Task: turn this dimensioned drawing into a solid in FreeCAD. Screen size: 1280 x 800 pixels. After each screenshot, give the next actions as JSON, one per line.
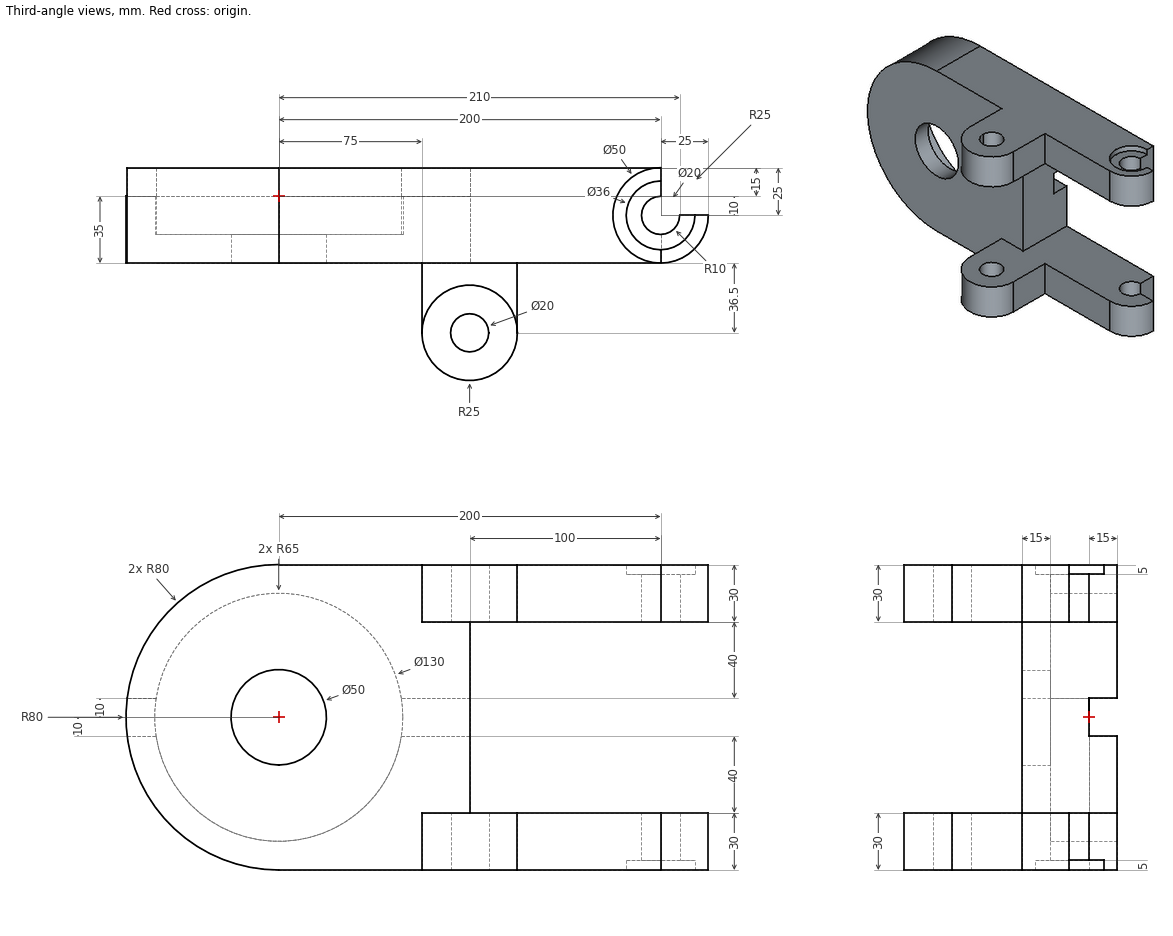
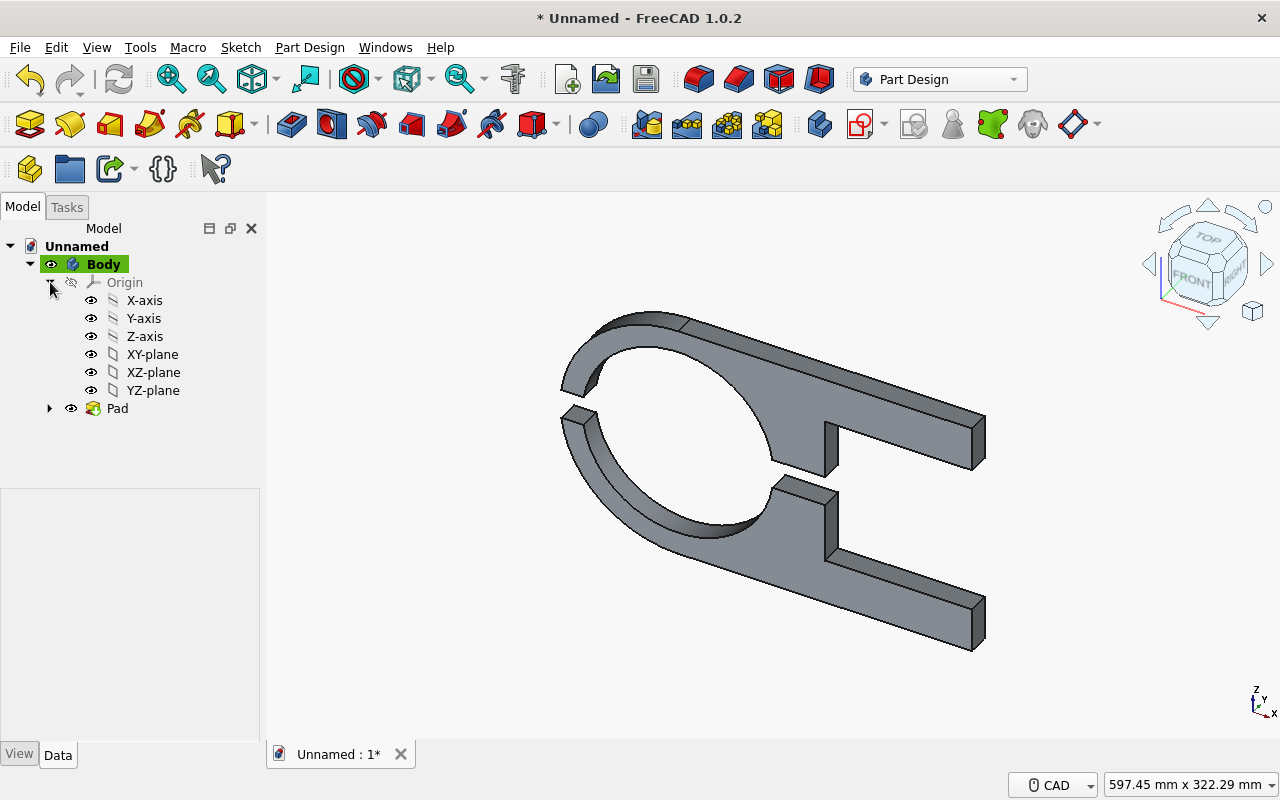
{"action": "left_click", "coordinate": [136, 372]}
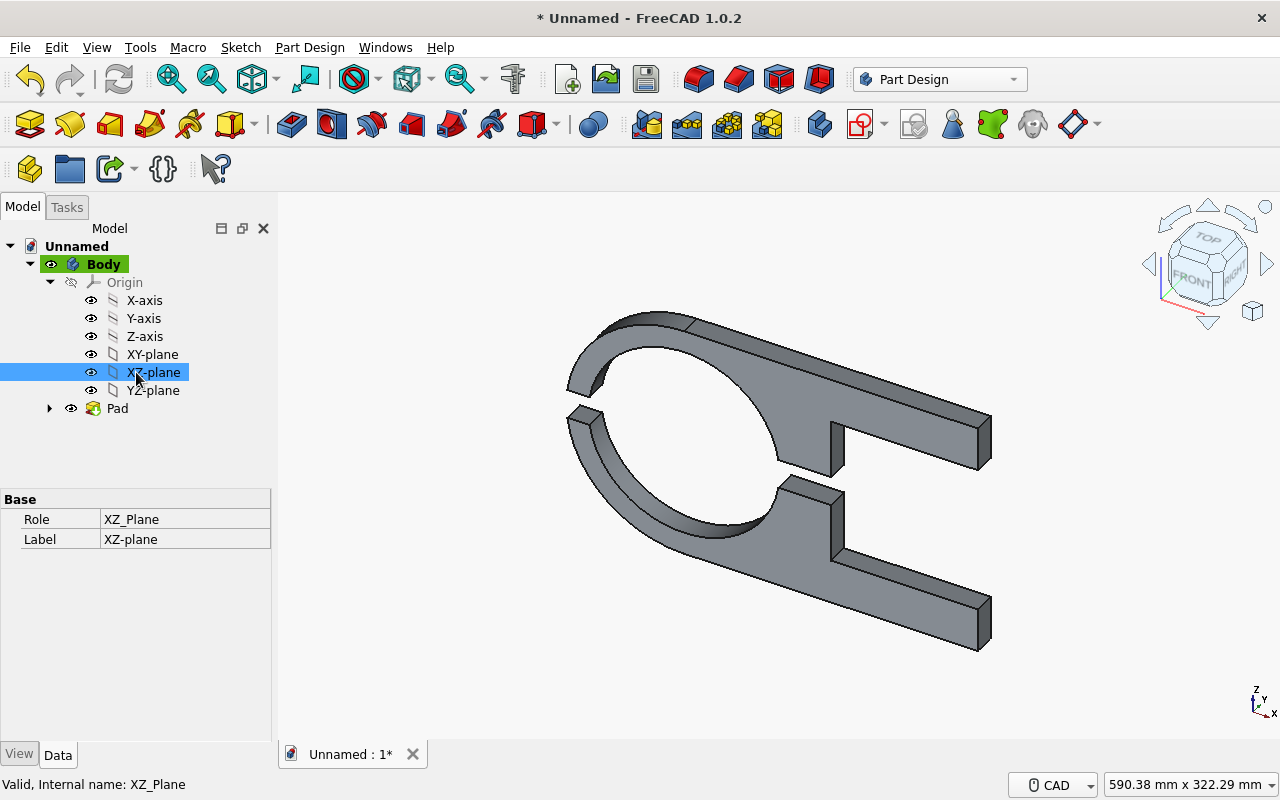
{"action": "left_click", "coordinate": [1074, 124]}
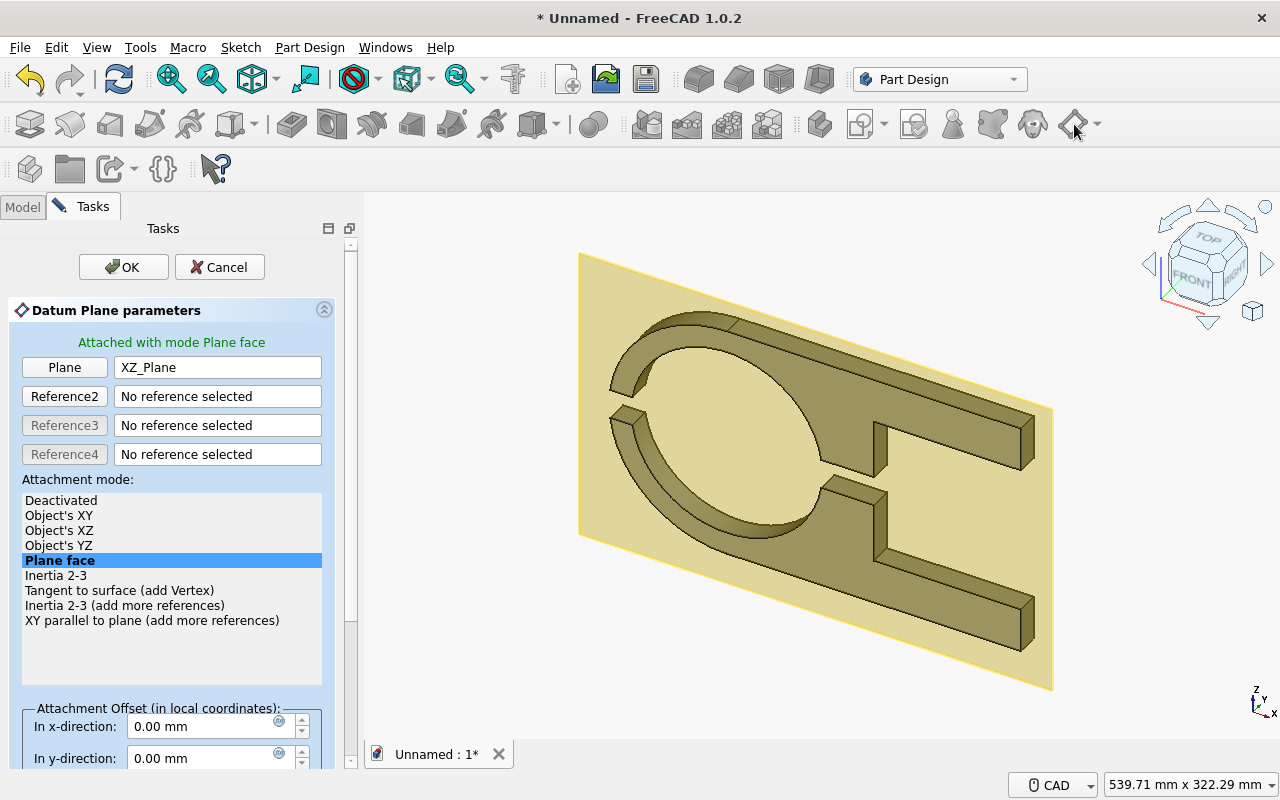
{"action": "scroll", "coordinate": [351, 503], "scroll_direction": "down", "scroll_amount": 2}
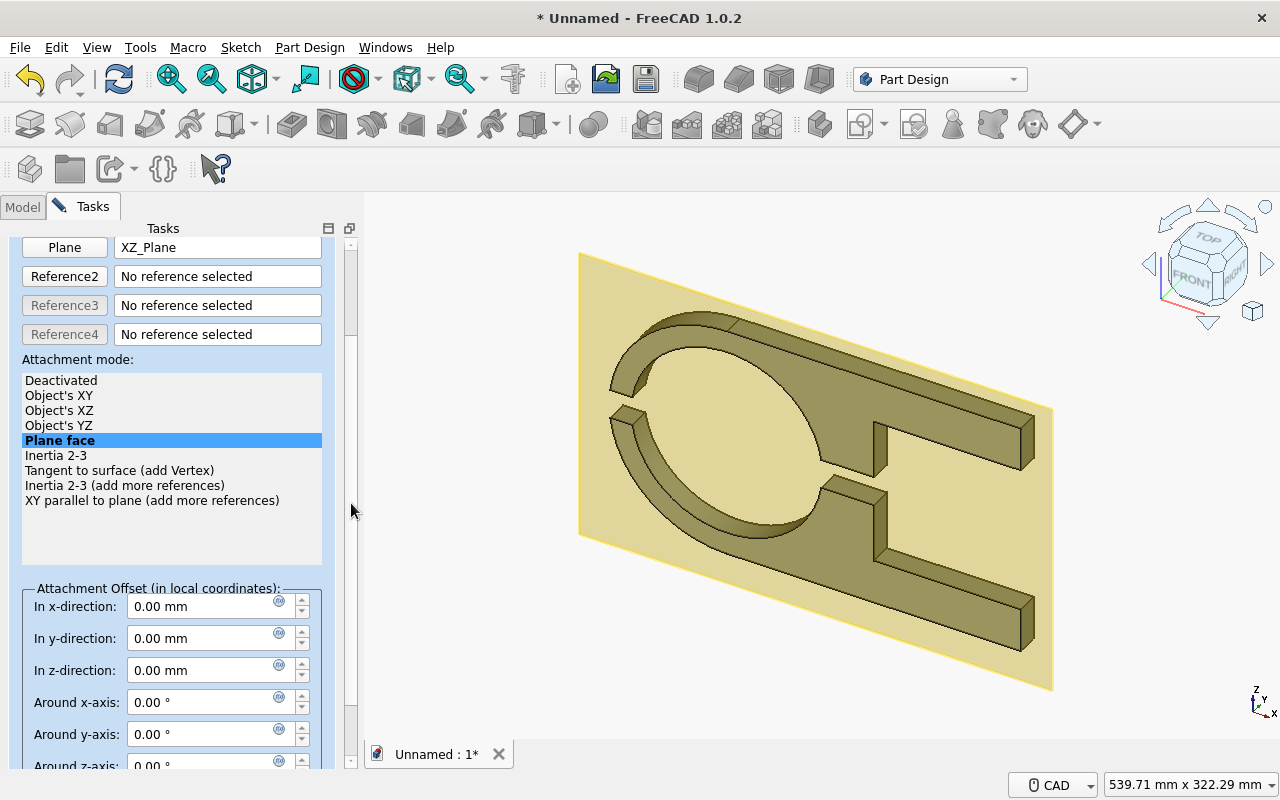
{"action": "triple_click", "coordinate": [210, 670]}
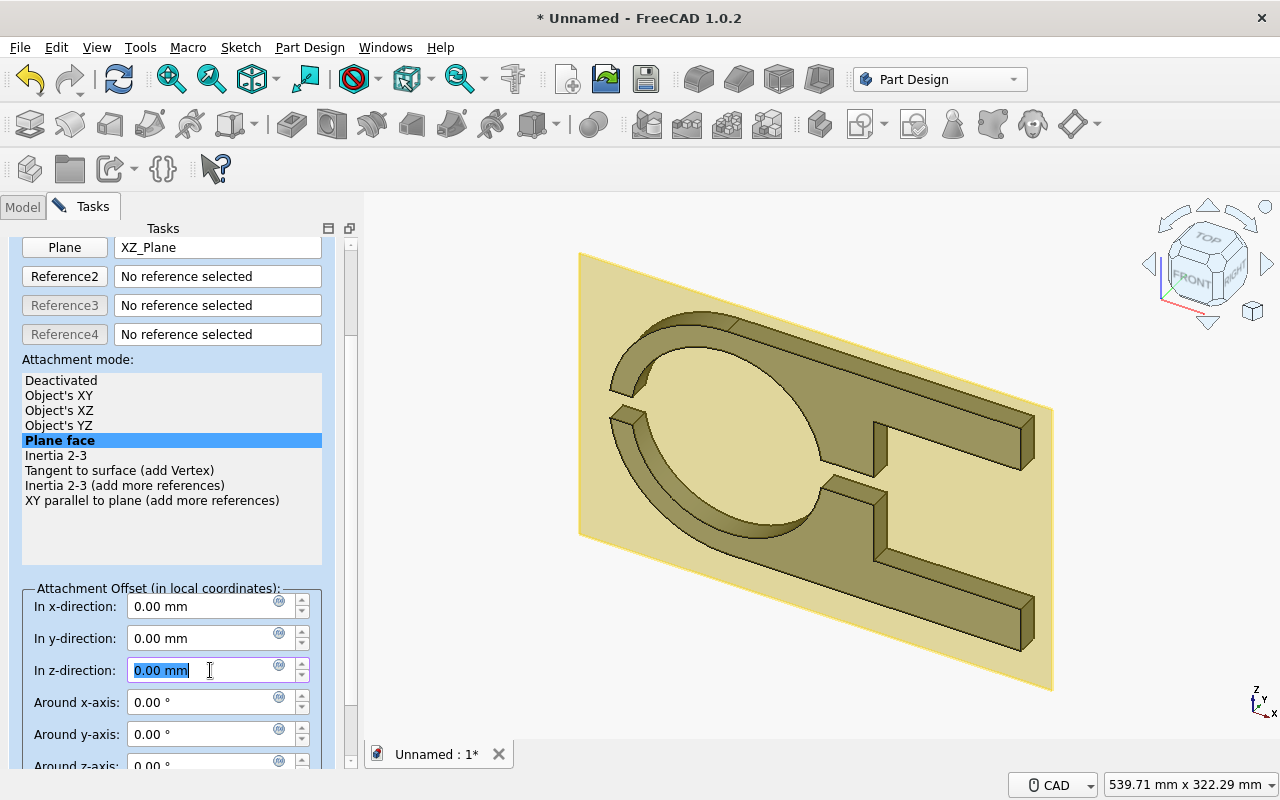
{"action": "type", "text": "35"}
{"action": "key", "text": "Tab"}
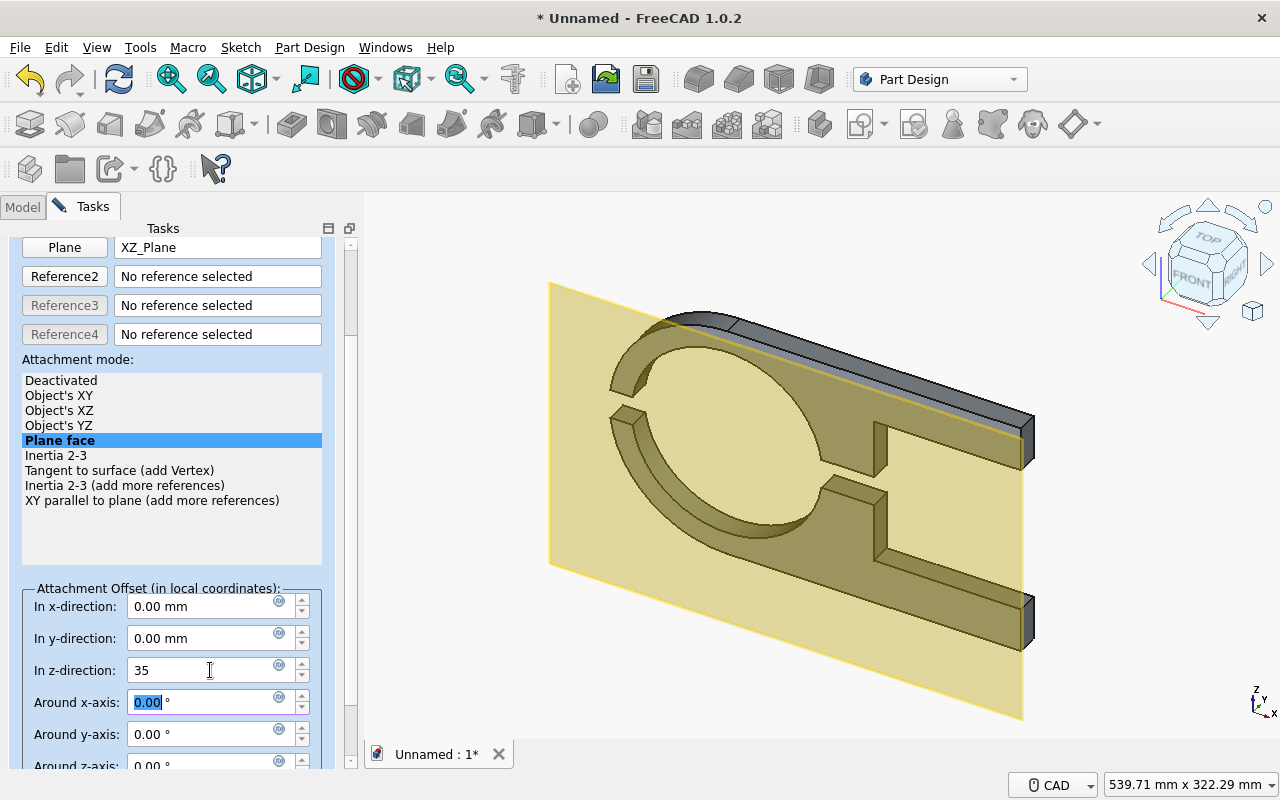
{"action": "scroll", "coordinate": [351, 503], "scroll_direction": "up", "scroll_amount": 3}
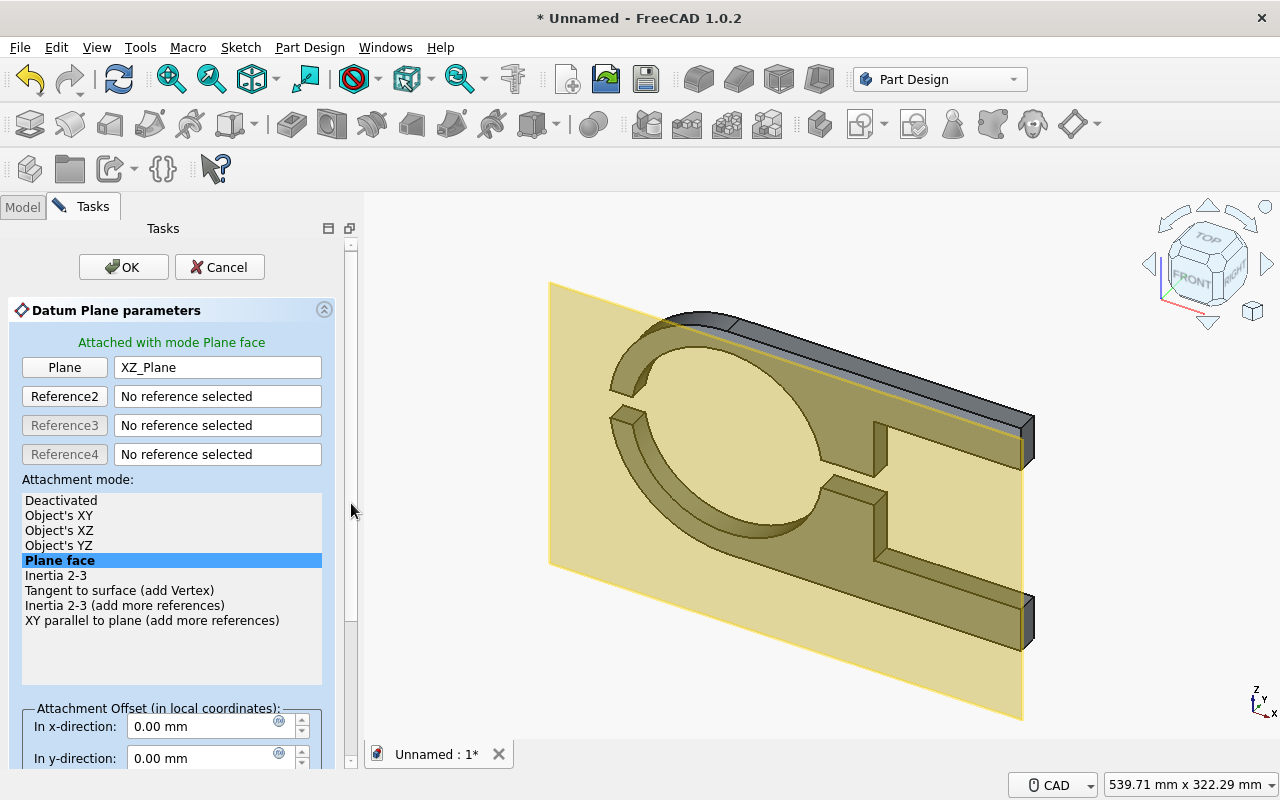
{"action": "left_click", "coordinate": [124, 267]}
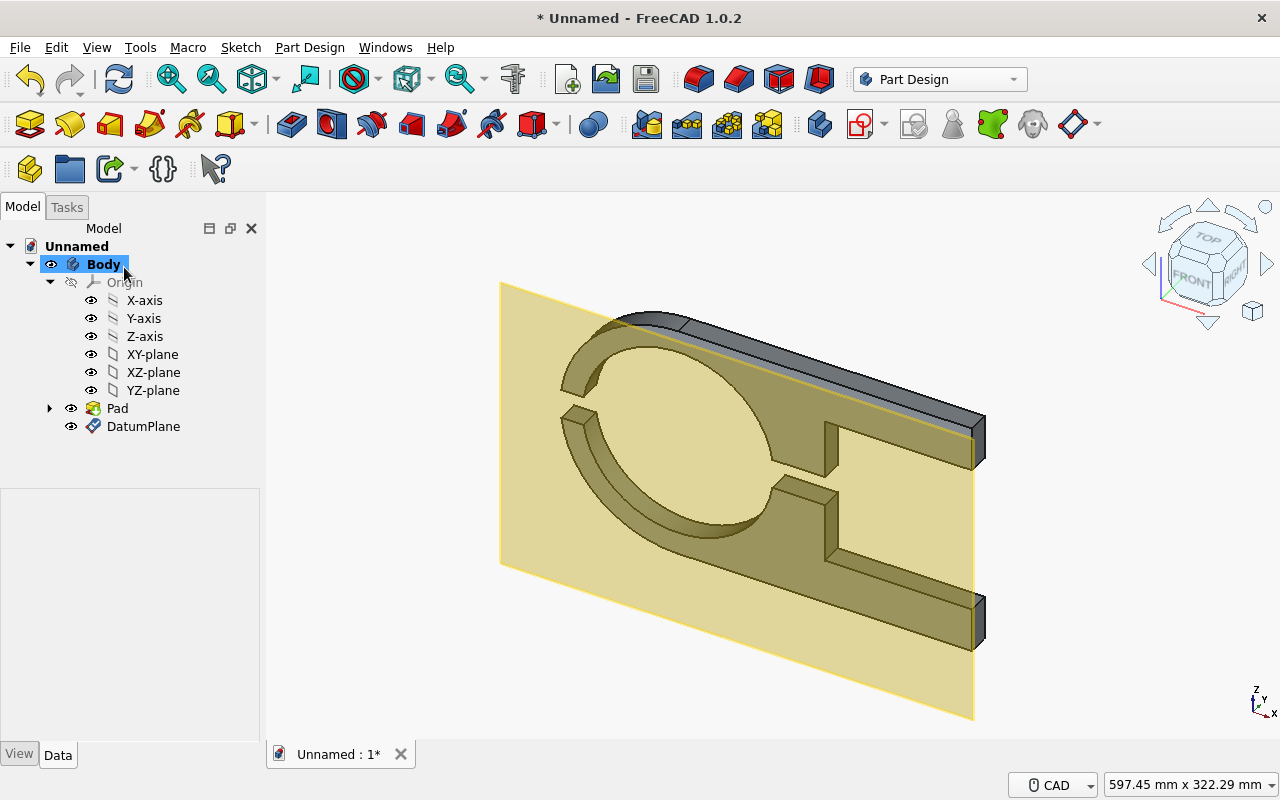
{"action": "left_click", "coordinate": [116, 426]}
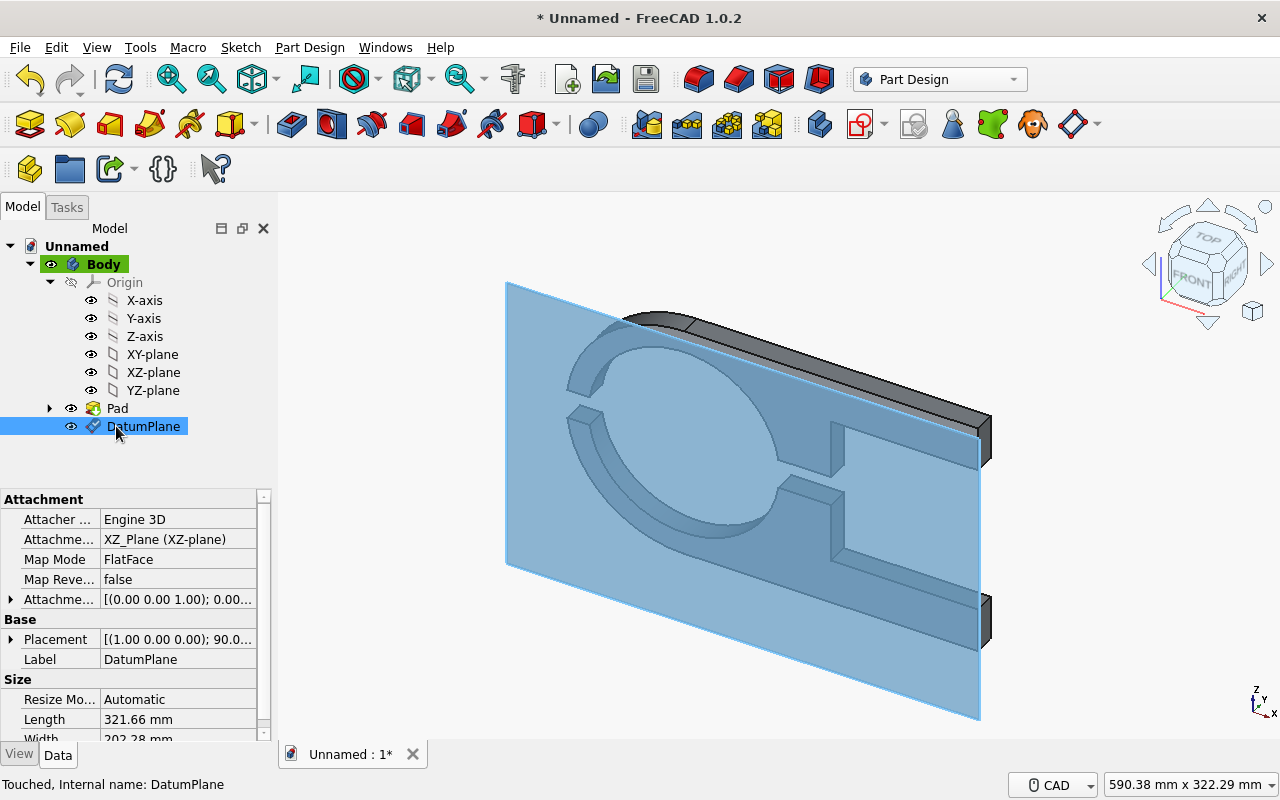
{"action": "left_click", "coordinate": [860, 124]}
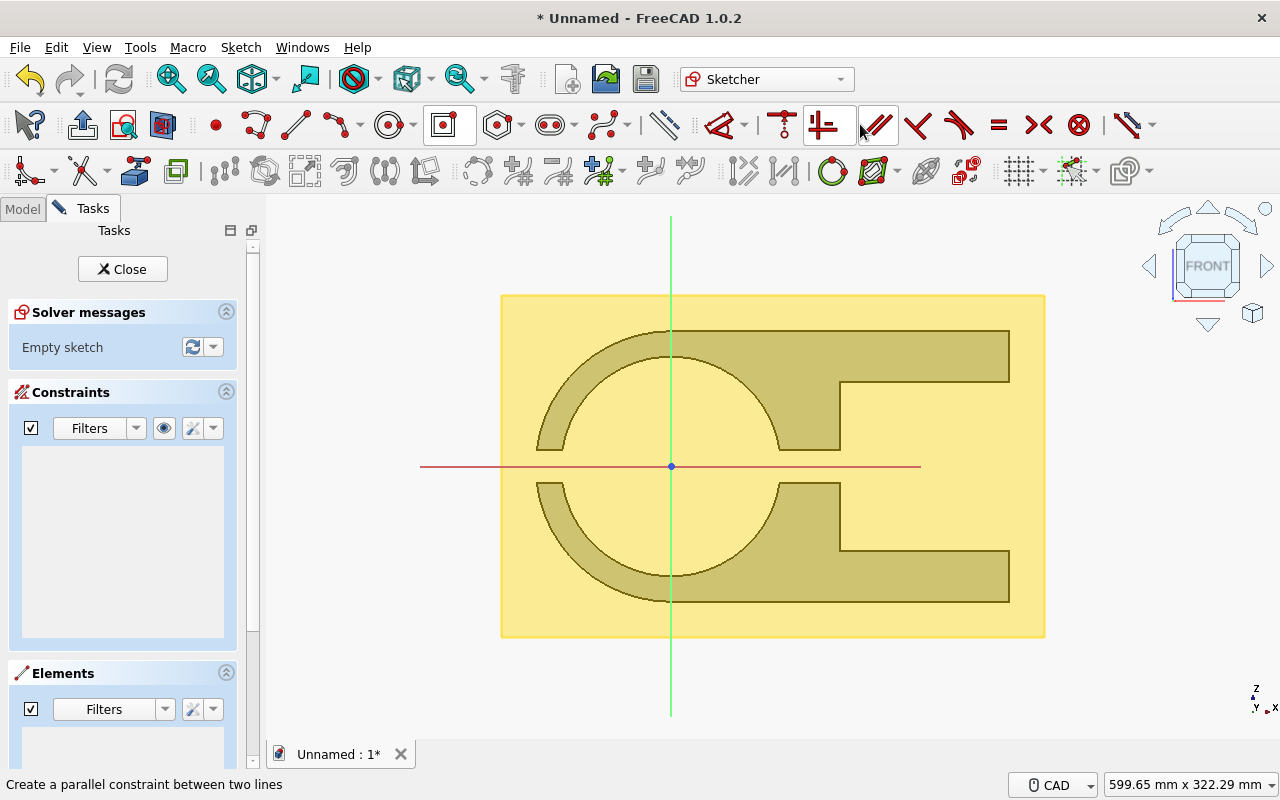
{"action": "left_click", "coordinate": [256, 126]}